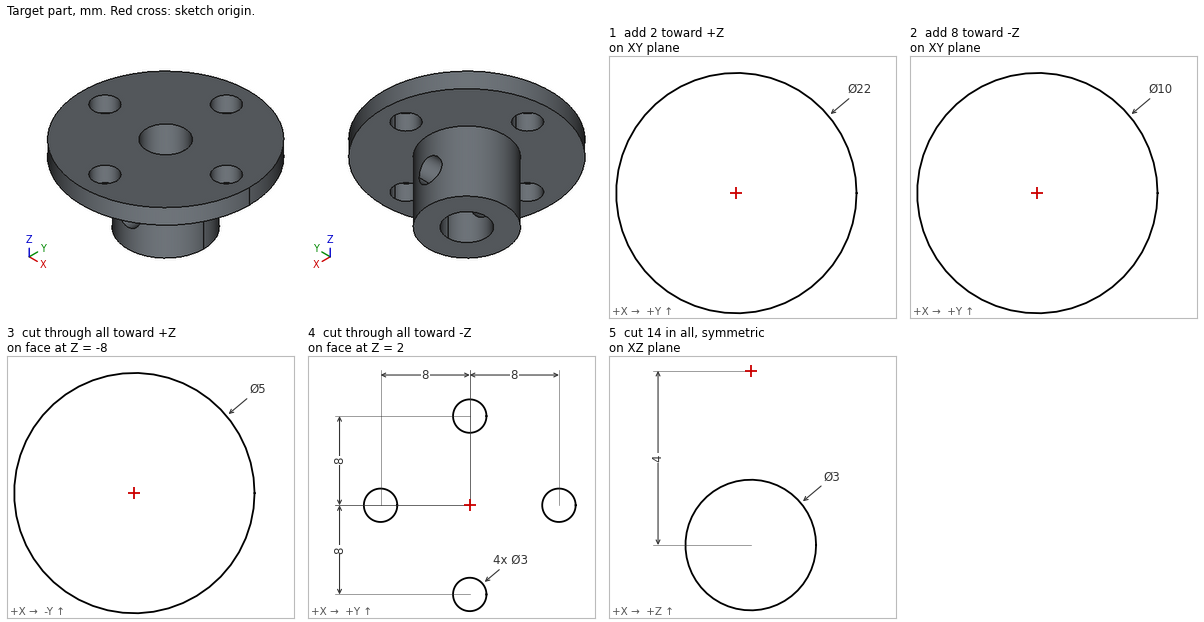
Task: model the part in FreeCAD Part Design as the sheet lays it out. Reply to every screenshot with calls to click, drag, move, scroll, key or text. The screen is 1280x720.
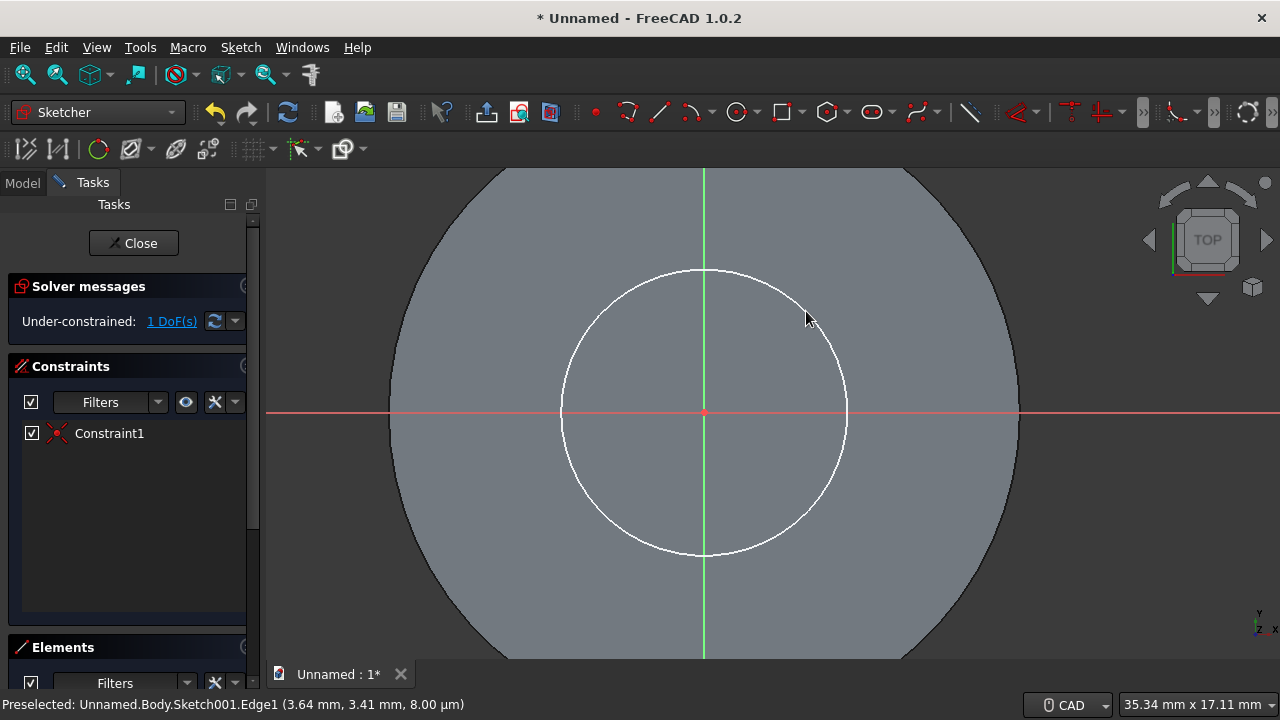
click(805, 311)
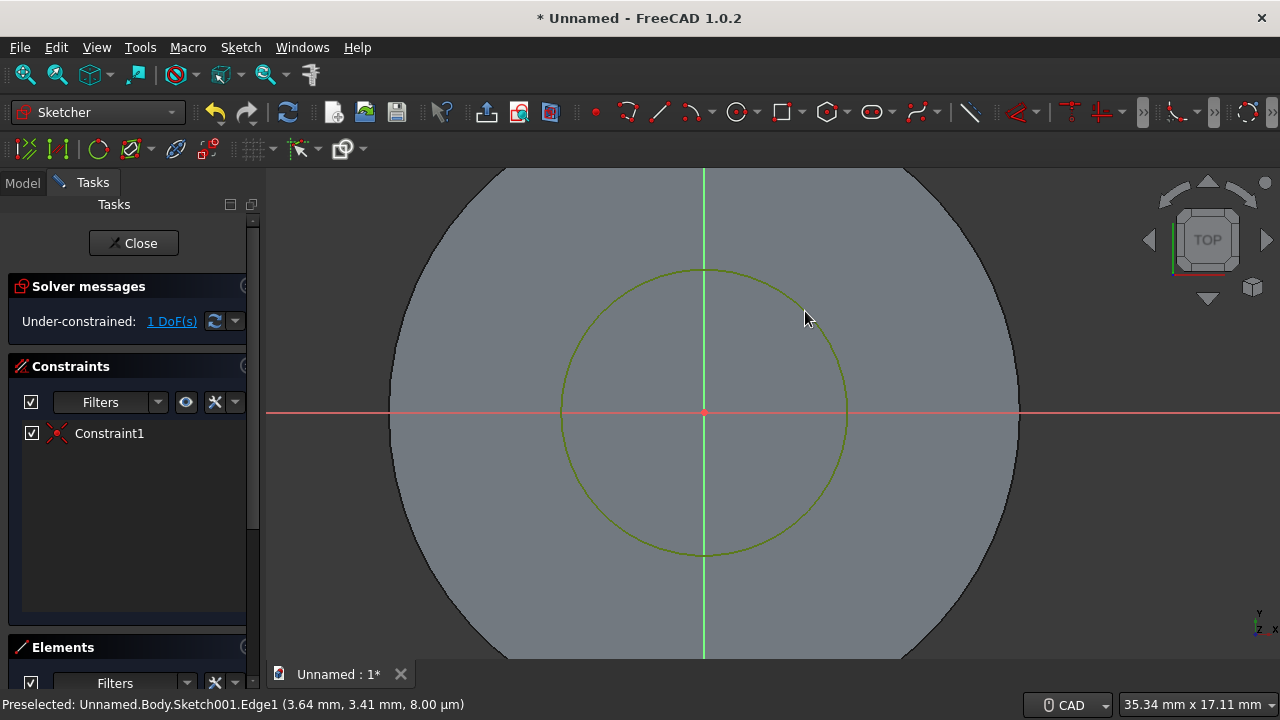
key(k)
key(o)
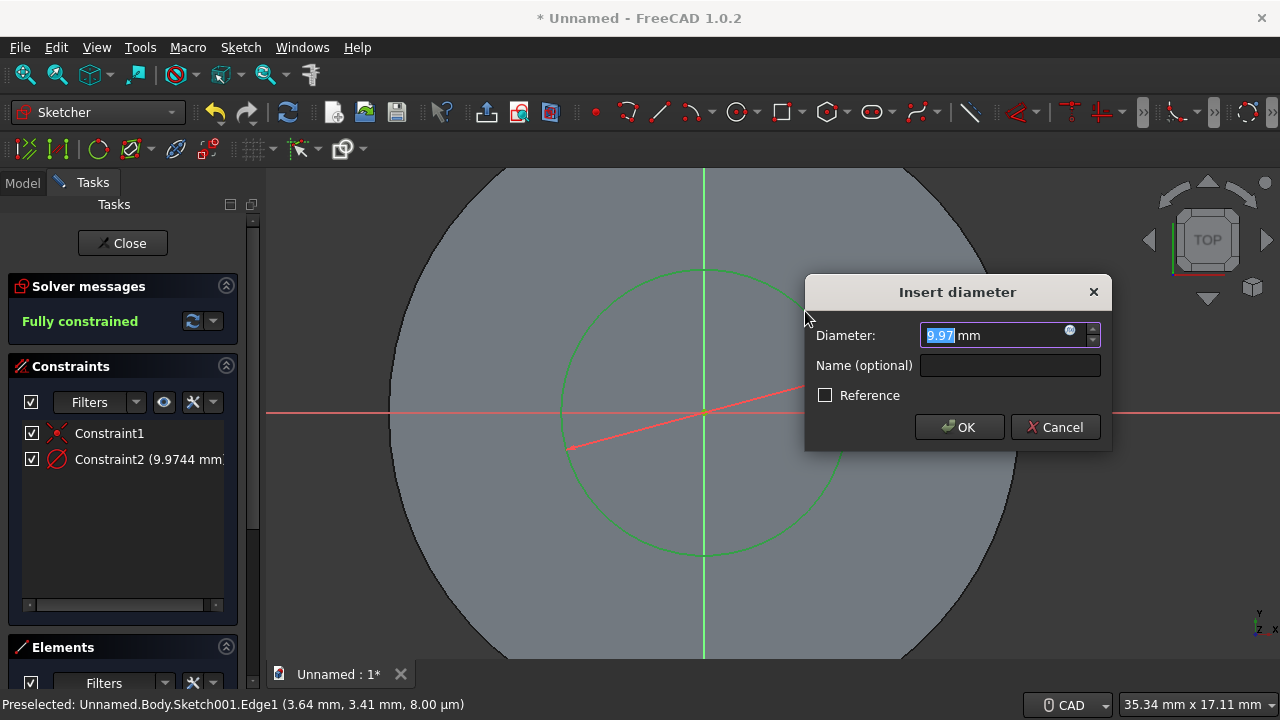
text(10)
key(Return)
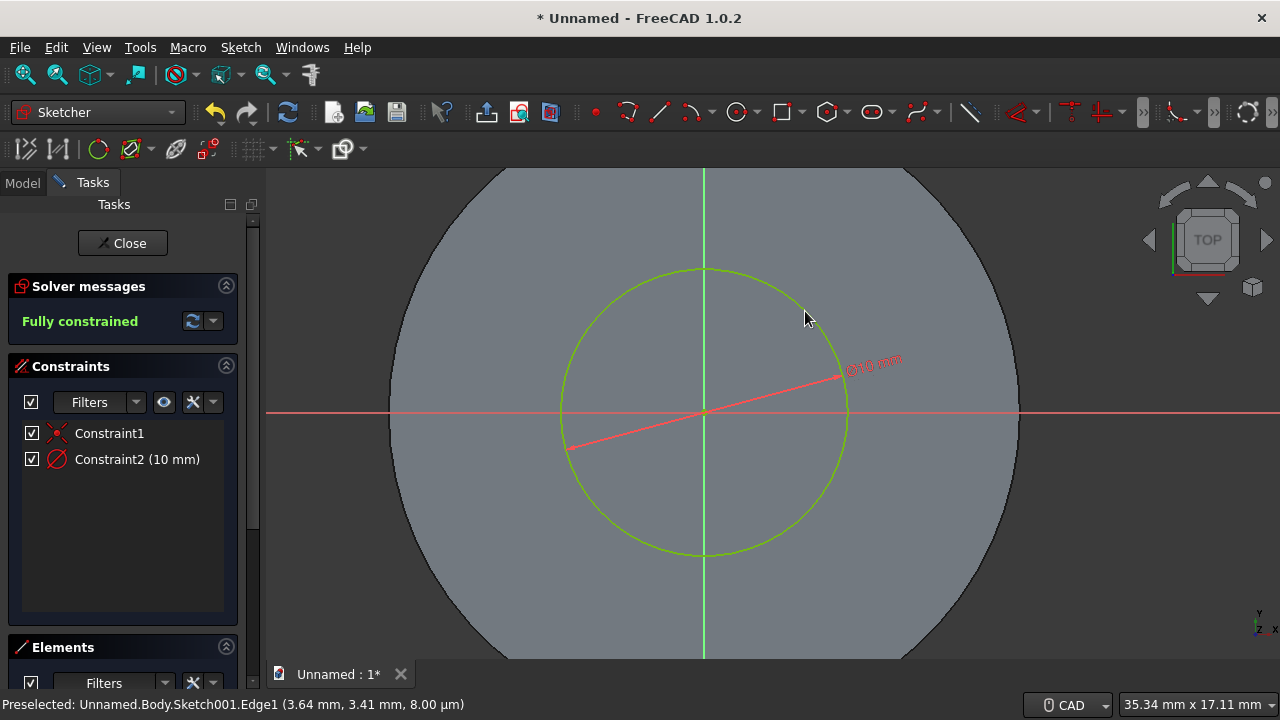
click(123, 243)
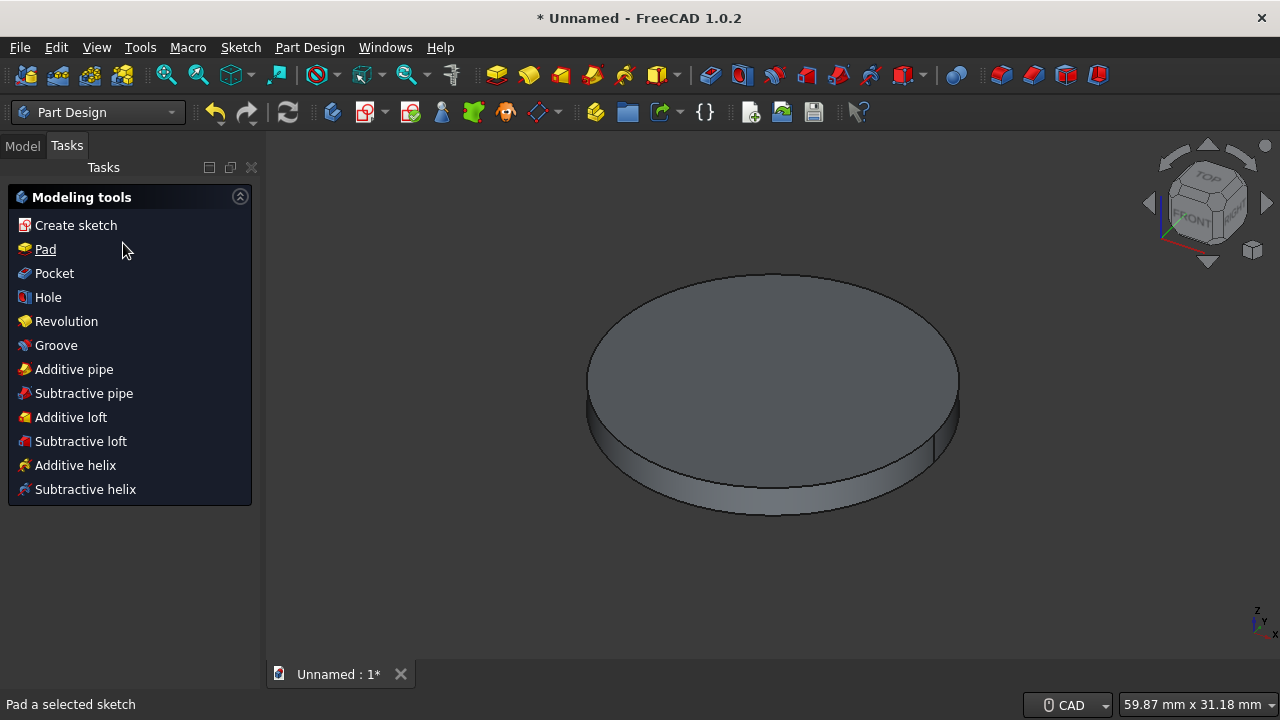
click(498, 76)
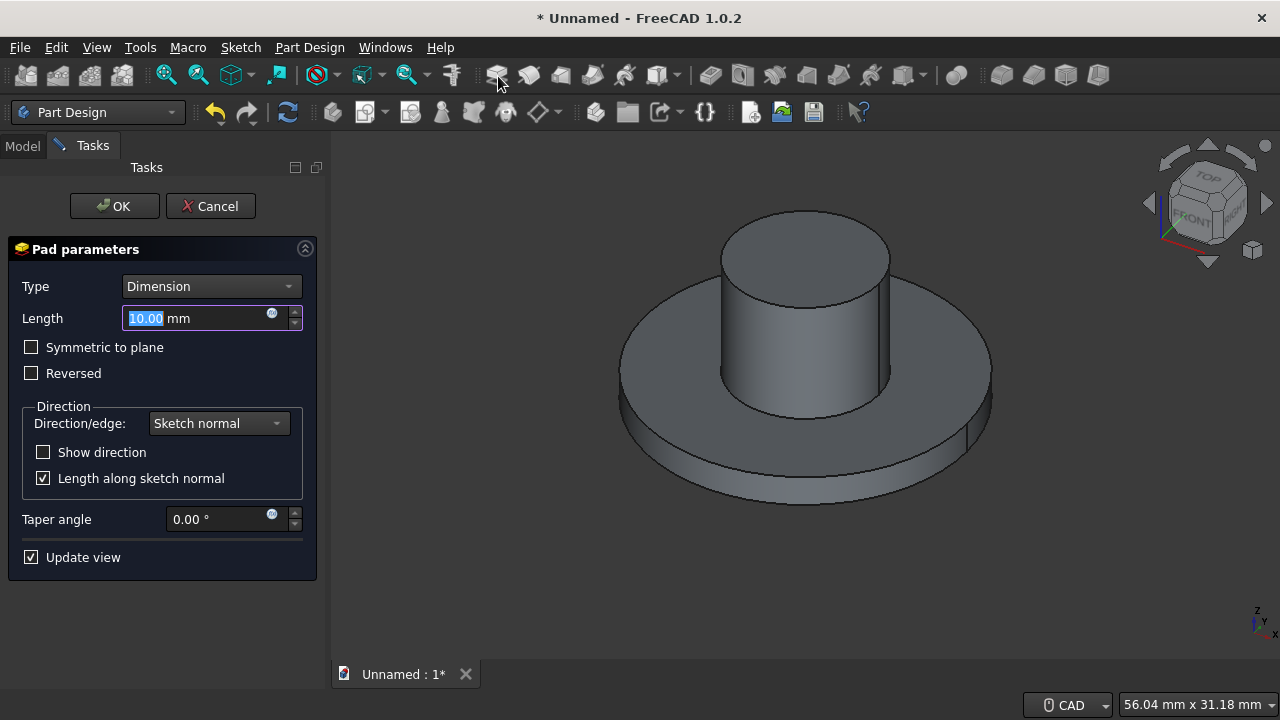
text(8)
key(Tab)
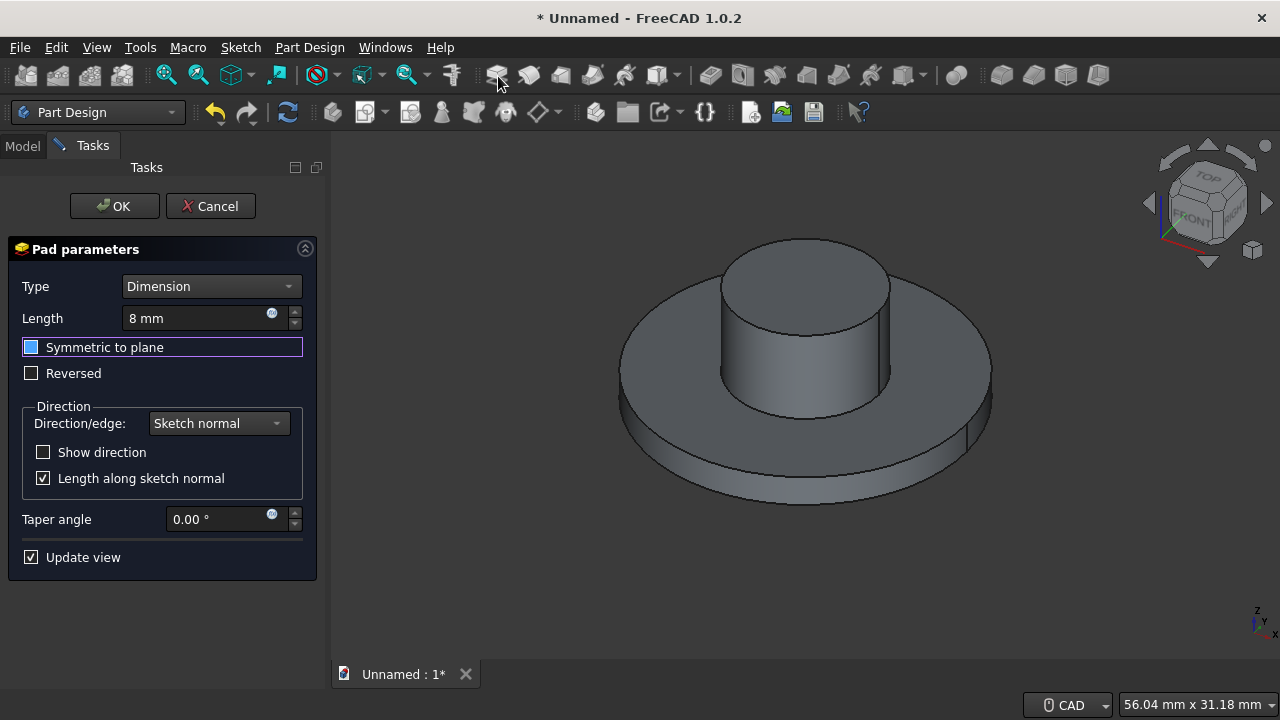
click(30, 373)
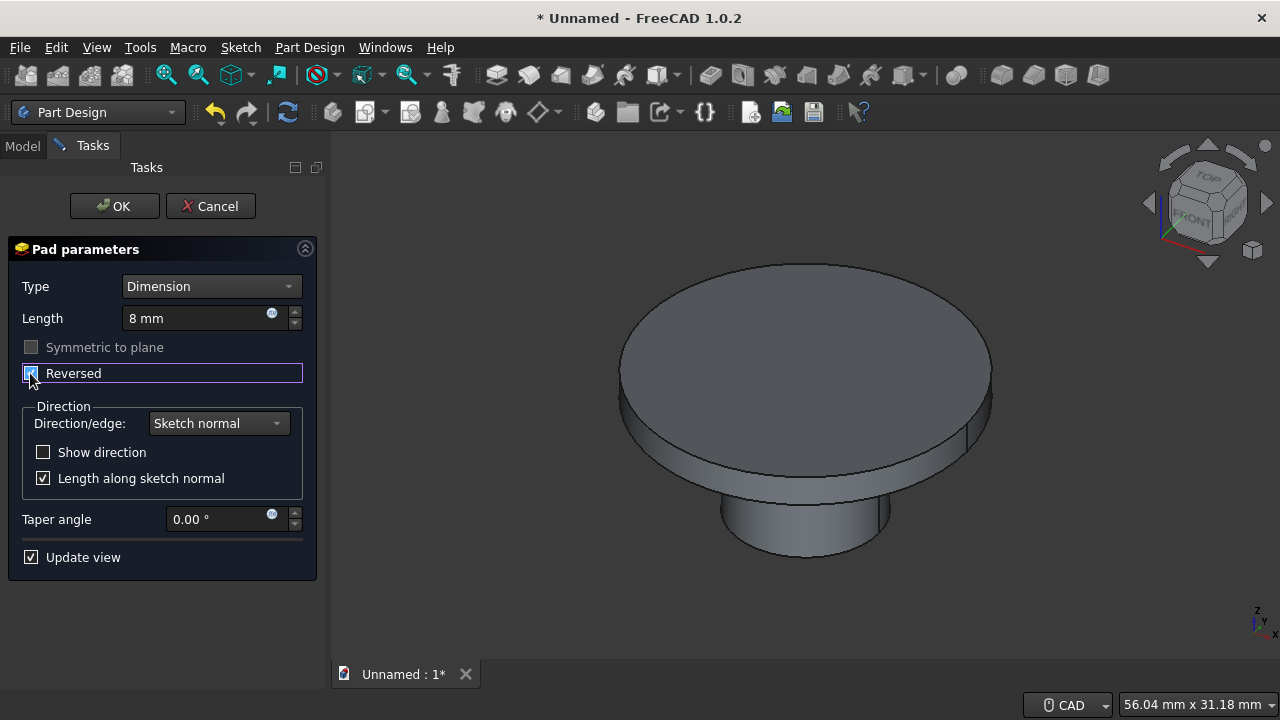
click(115, 206)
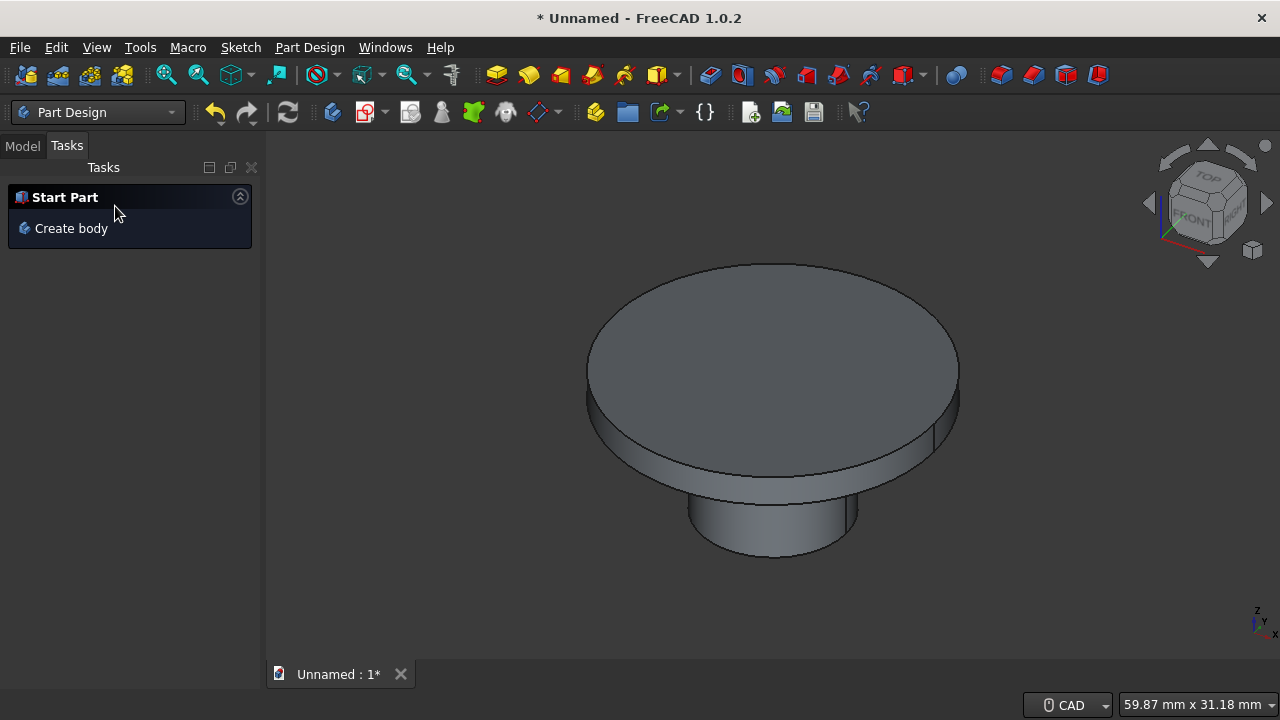
key(5)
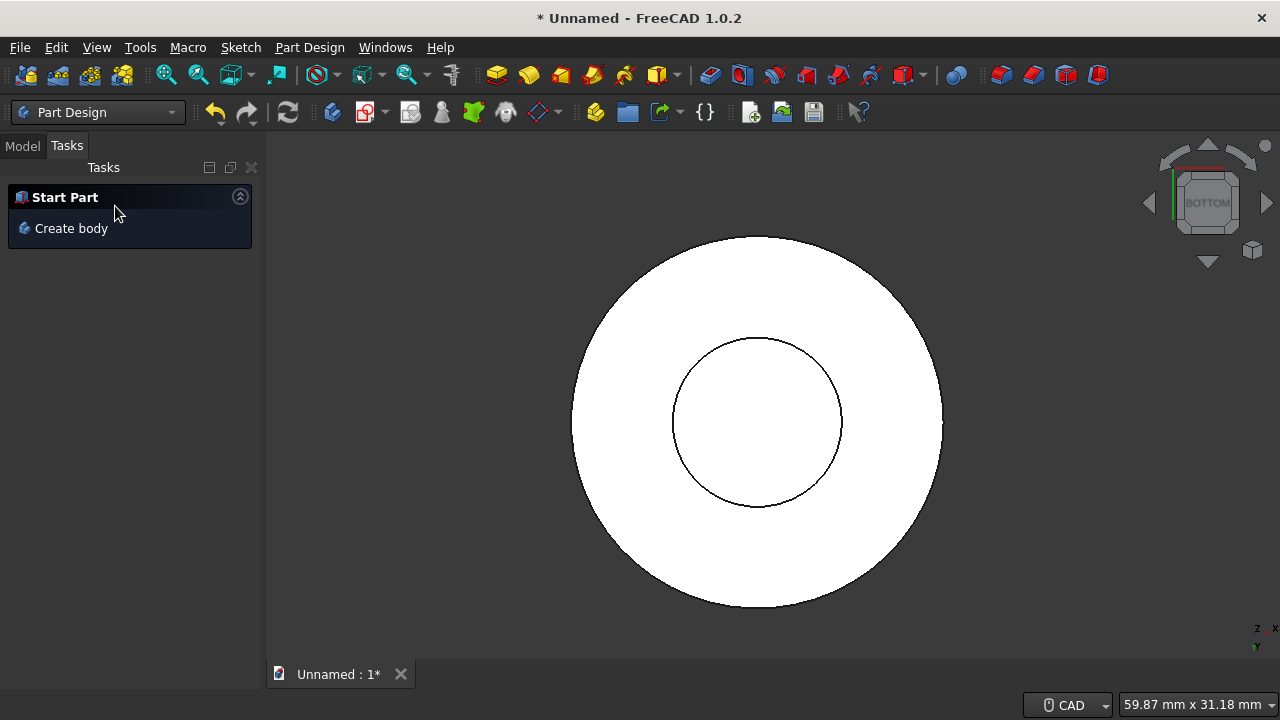
click(757, 421)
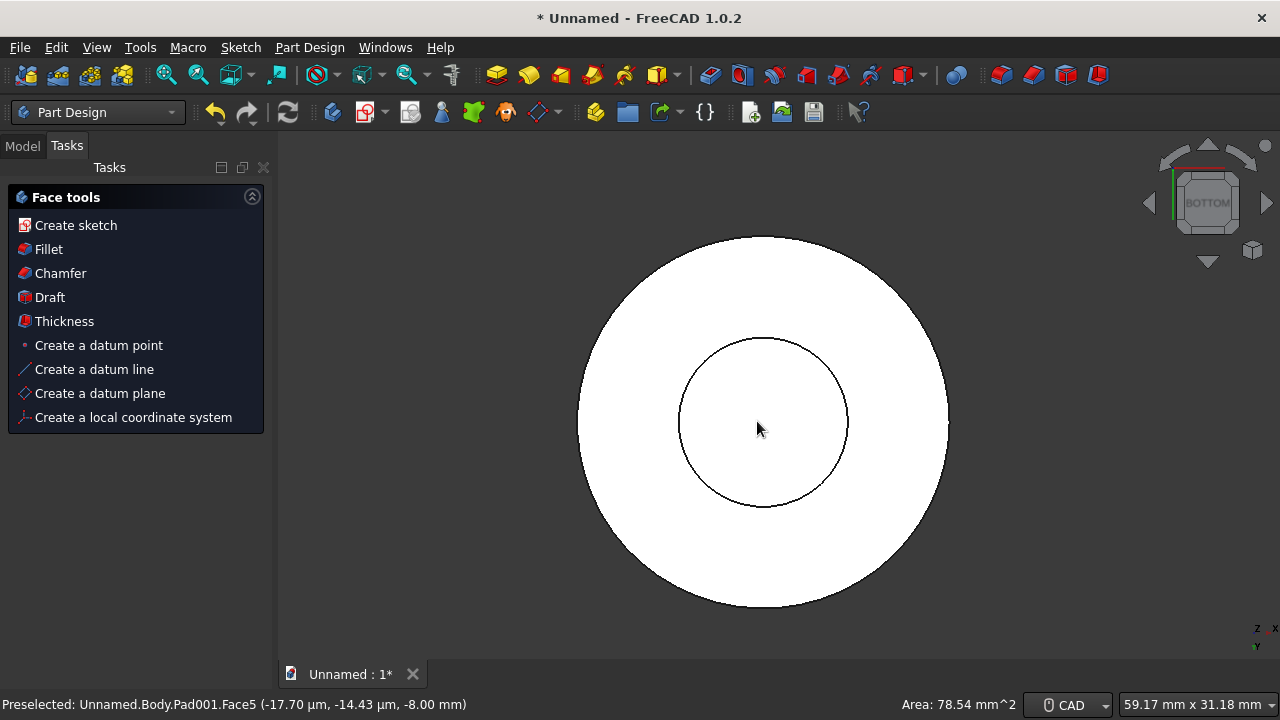
click(366, 112)